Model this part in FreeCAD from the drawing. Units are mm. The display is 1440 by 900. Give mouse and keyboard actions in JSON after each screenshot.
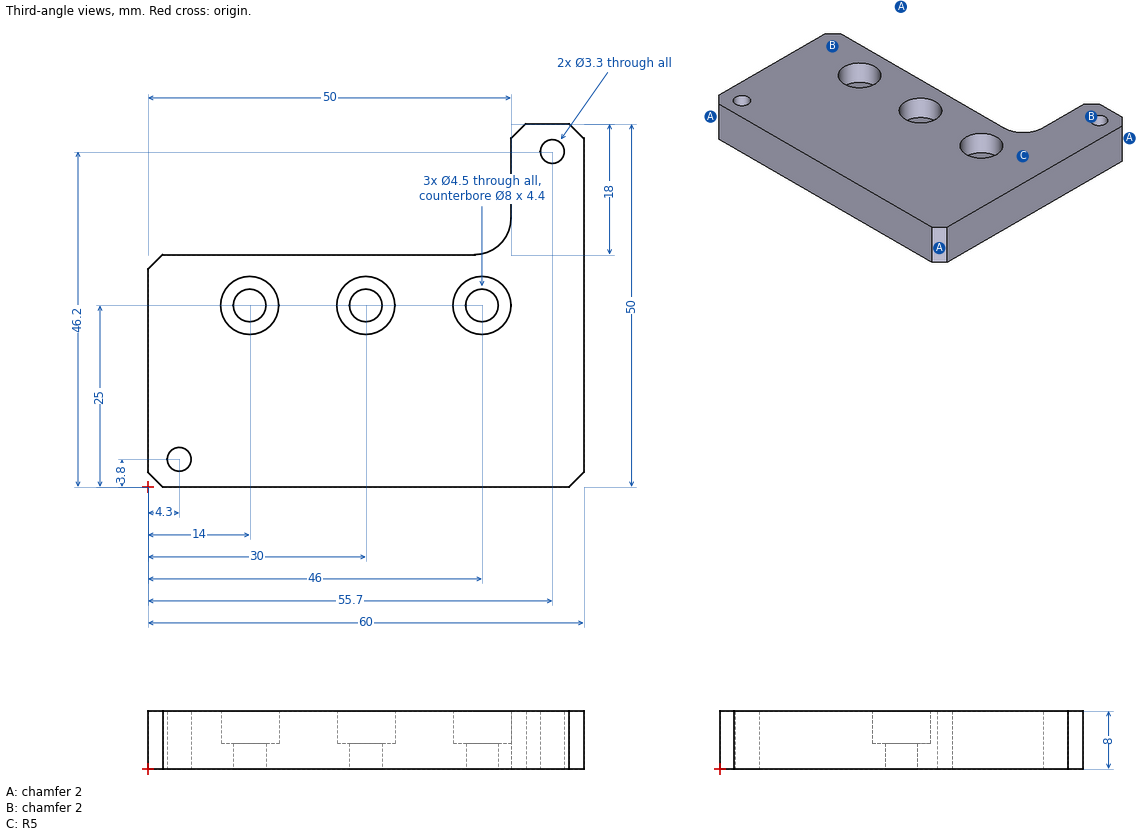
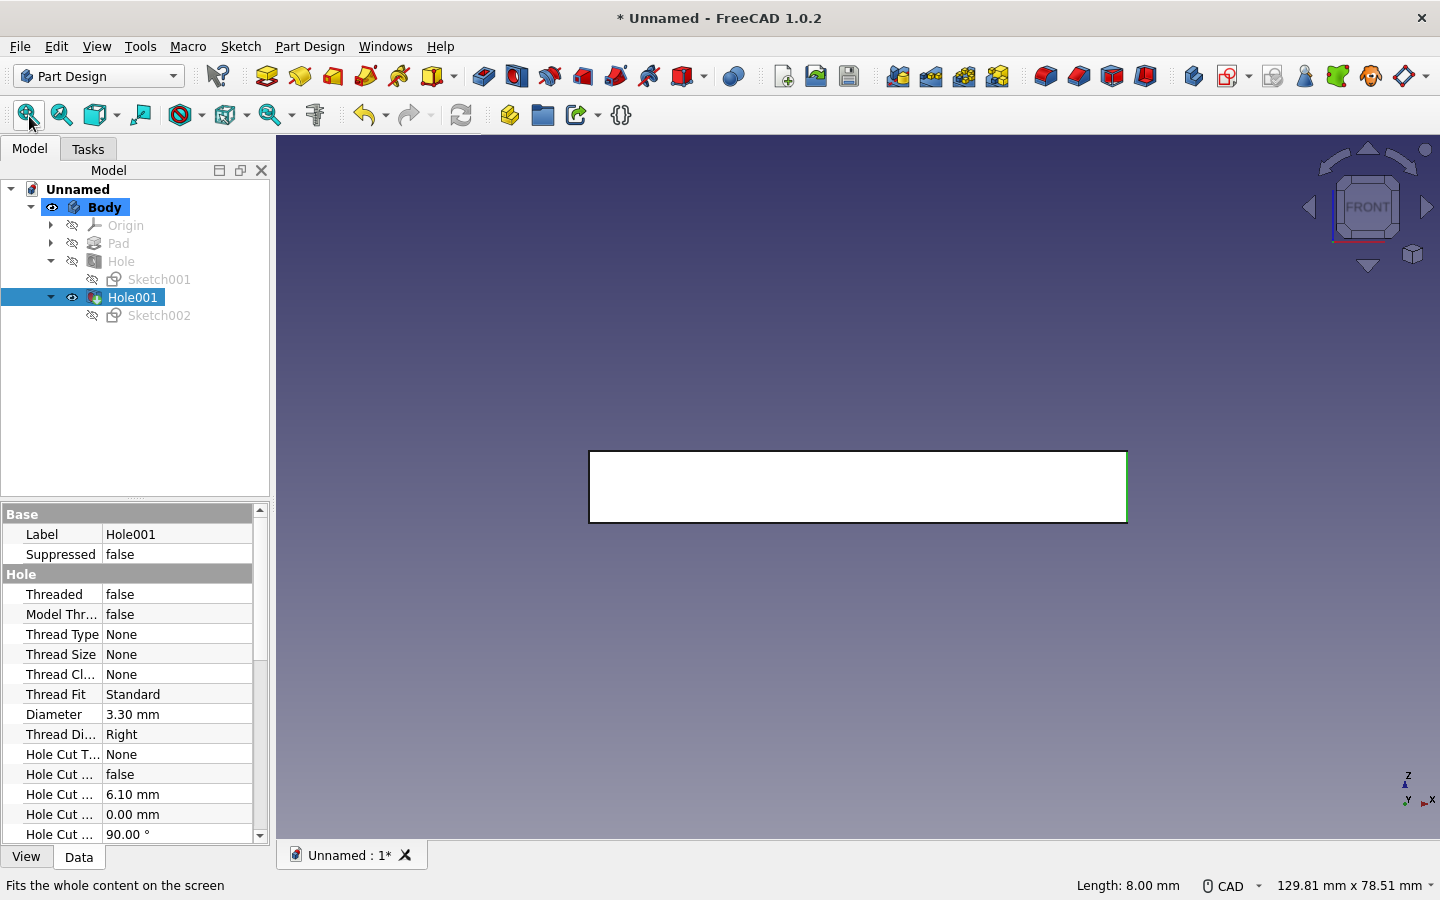
{"action": "left_click", "coordinate": [589, 486], "text": "ctrl"}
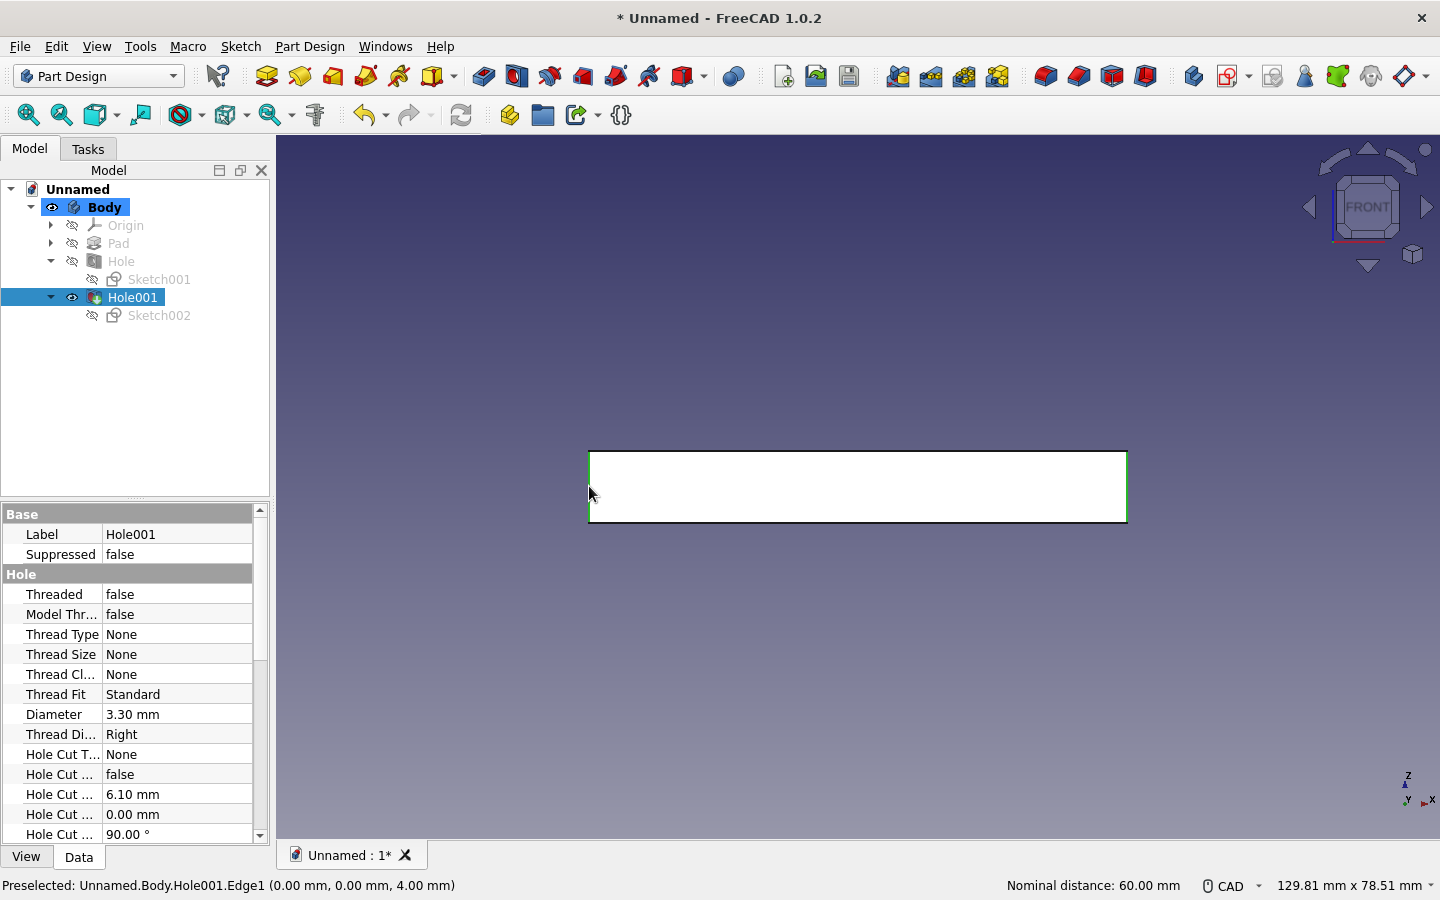
{"action": "key", "text": "3"}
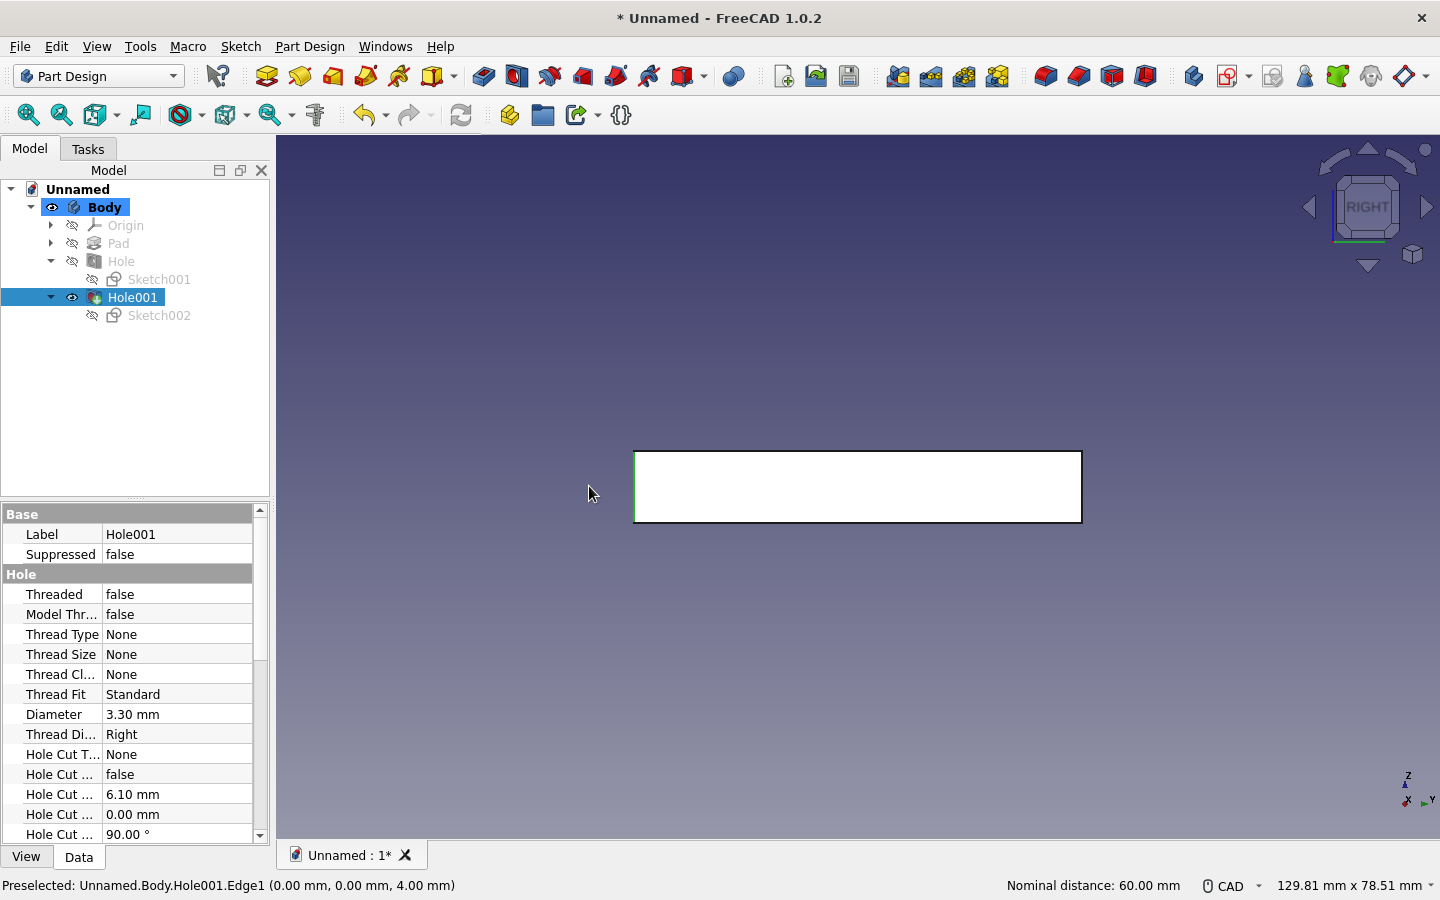
{"action": "left_click", "coordinate": [29, 116]}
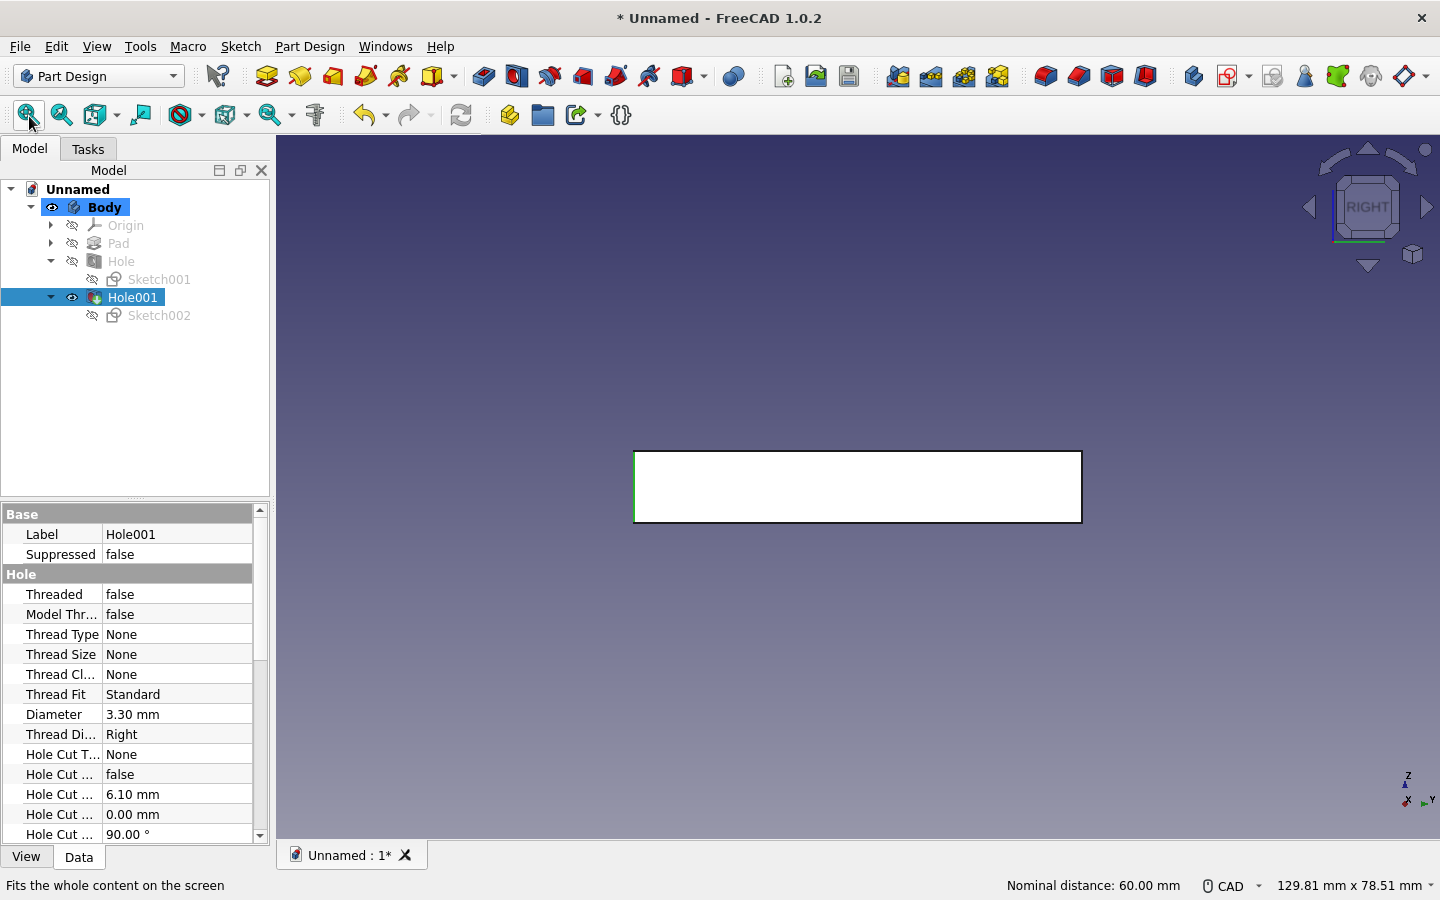
{"action": "left_click", "coordinate": [1082, 486], "text": "ctrl"}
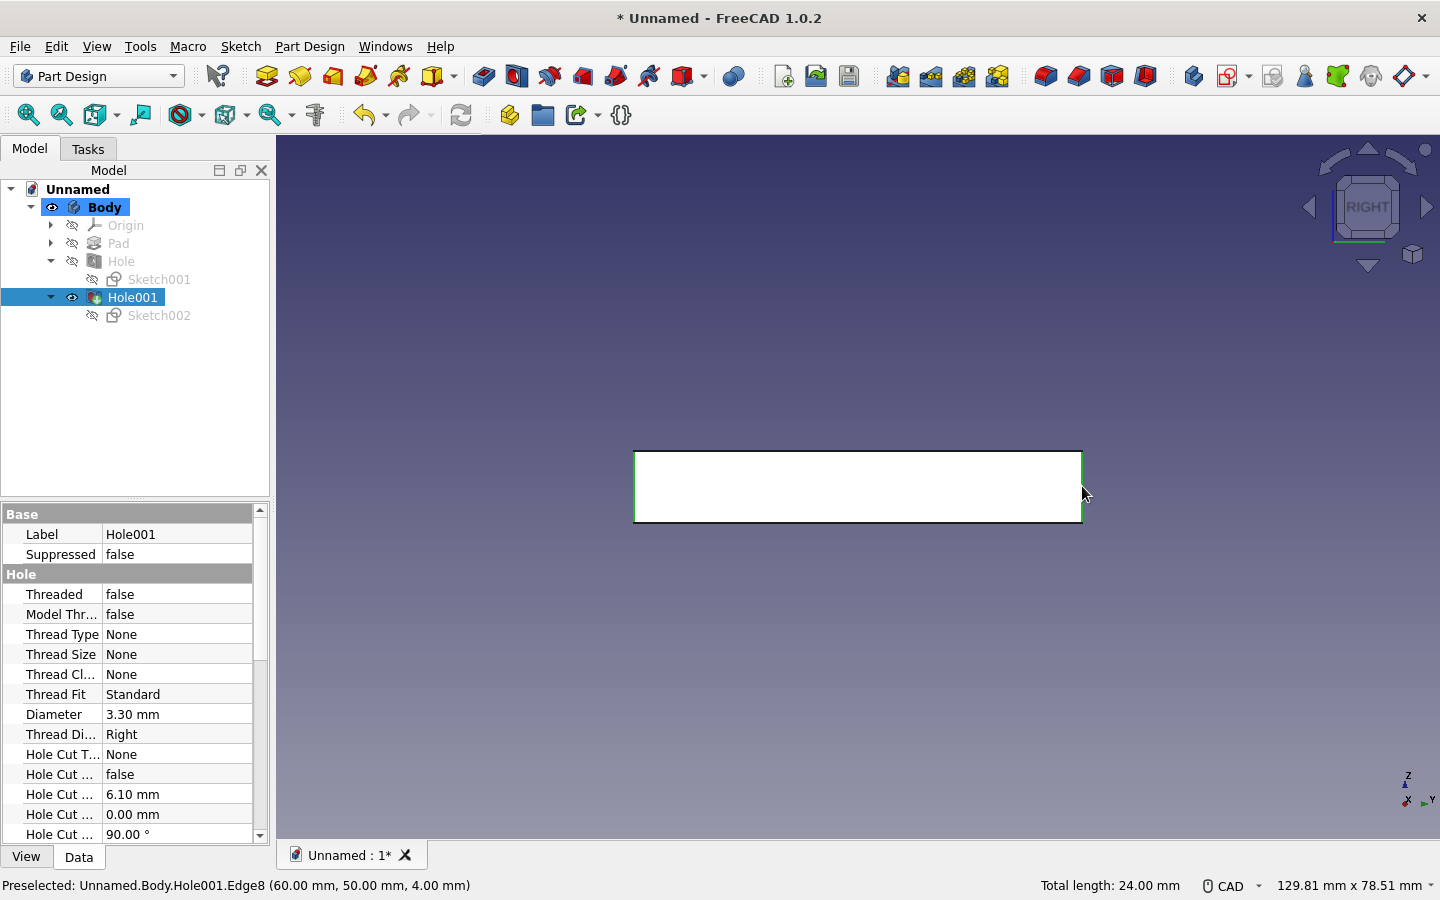
{"action": "key", "text": "5"}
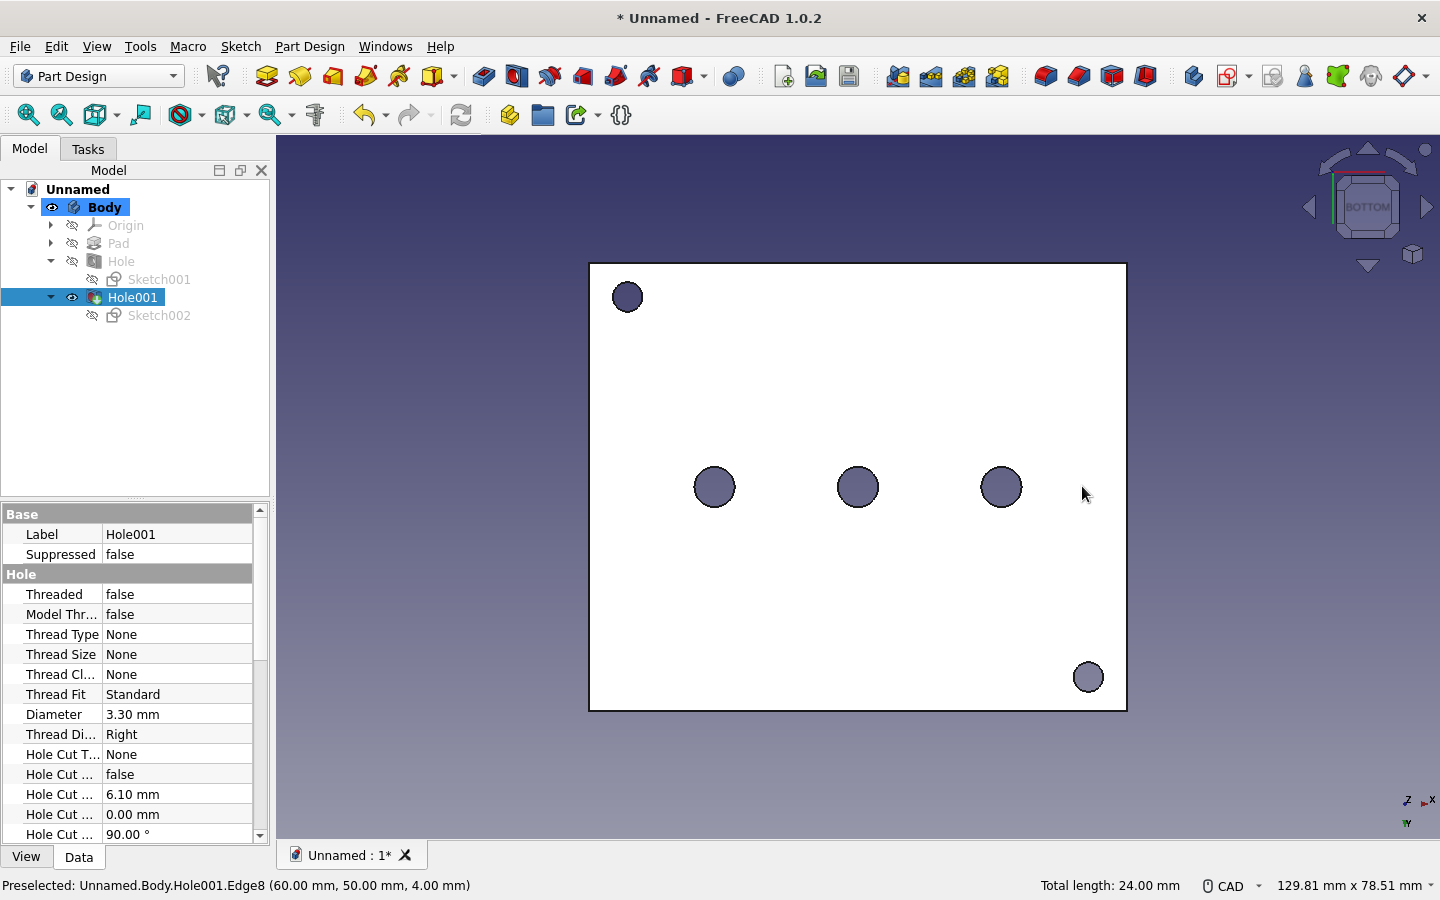
{"action": "key", "text": "4"}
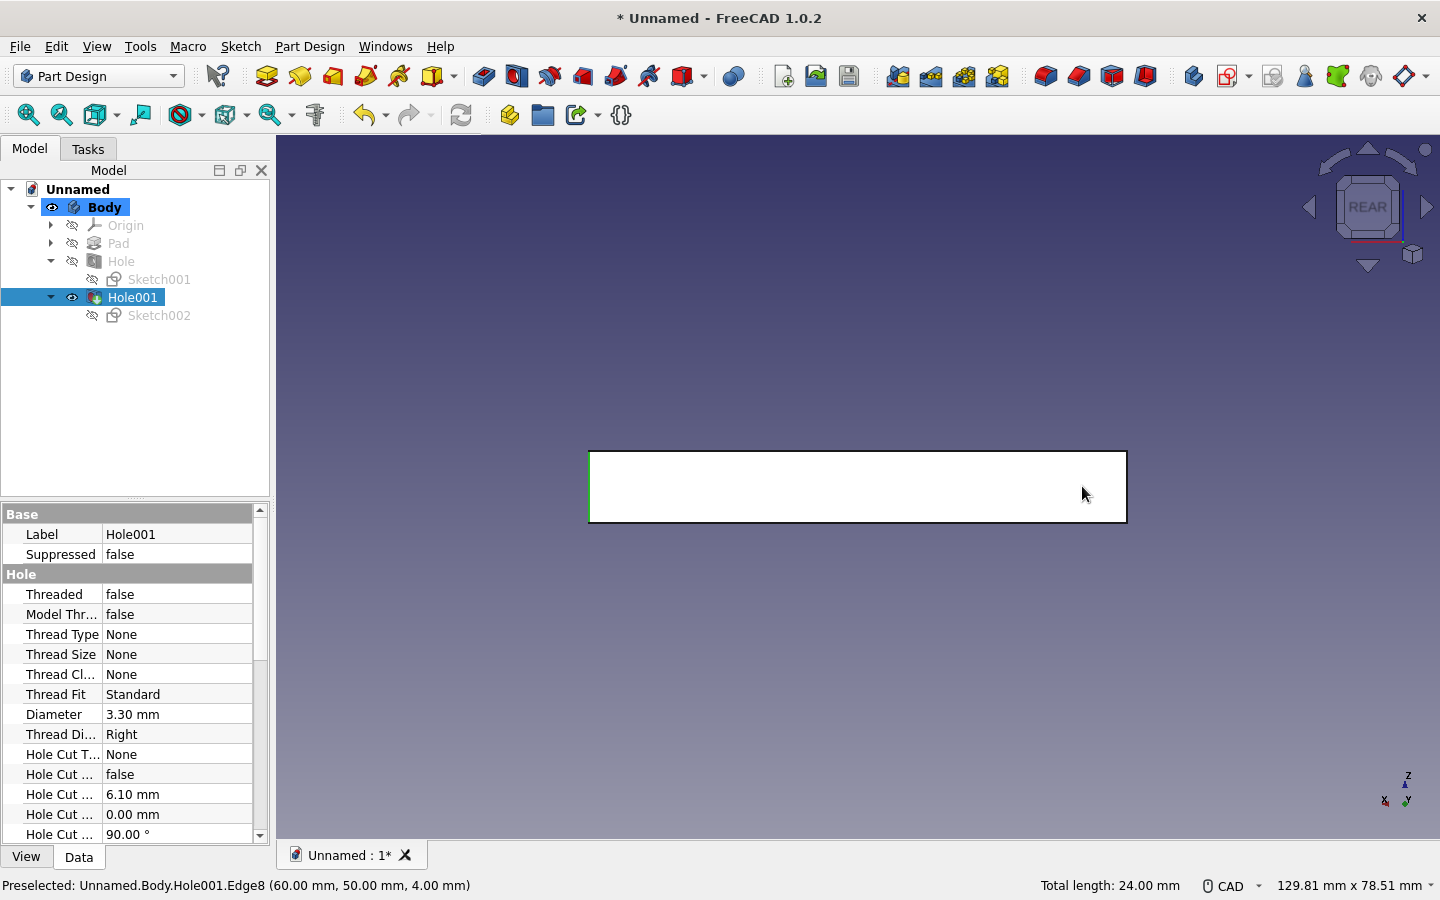
{"action": "left_click", "coordinate": [1127, 486], "text": "ctrl"}